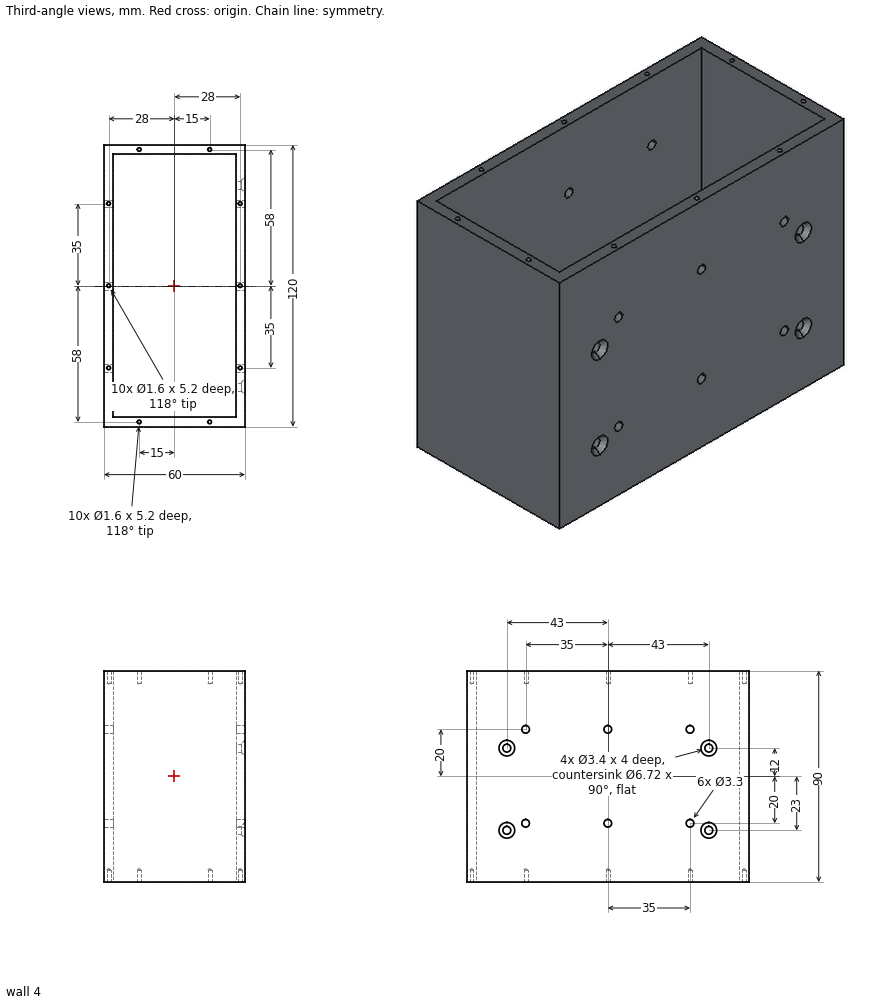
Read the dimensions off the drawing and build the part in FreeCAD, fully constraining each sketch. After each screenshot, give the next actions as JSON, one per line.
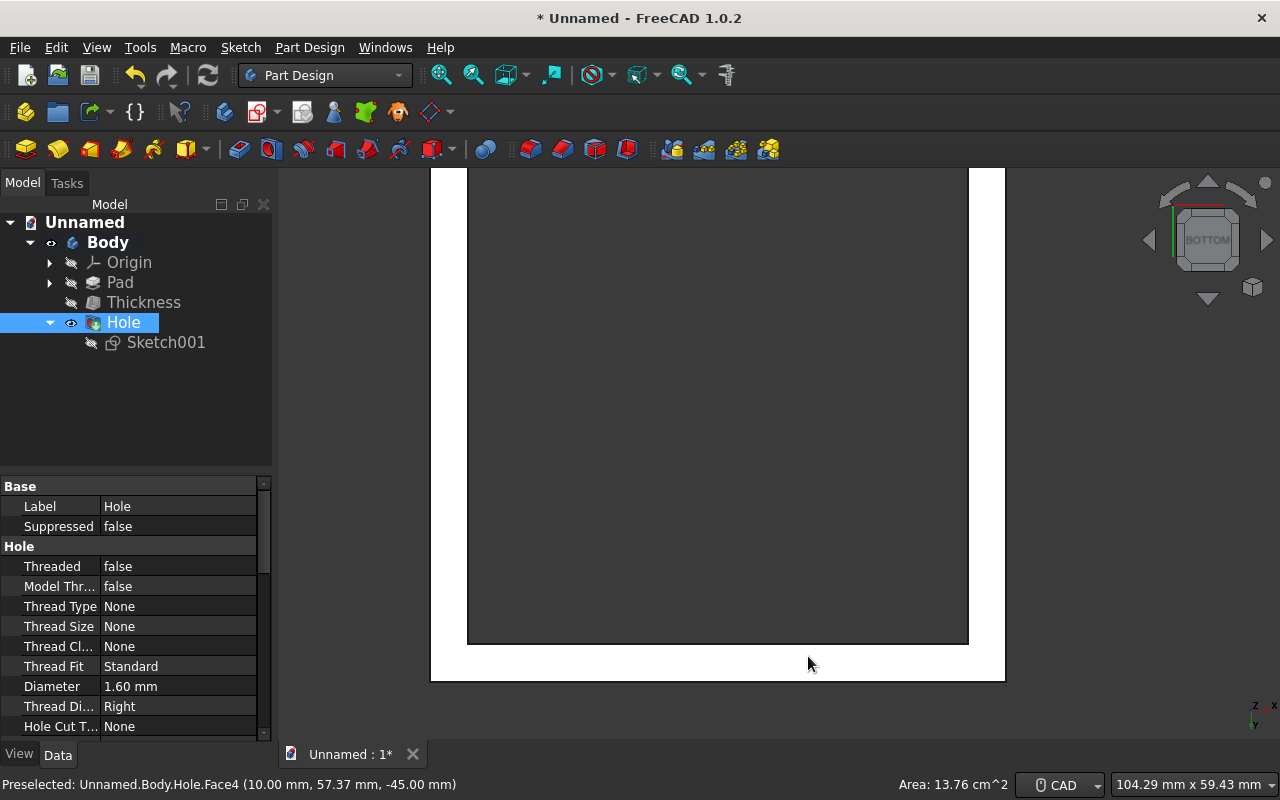
{"action": "left_click", "coordinate": [258, 112]}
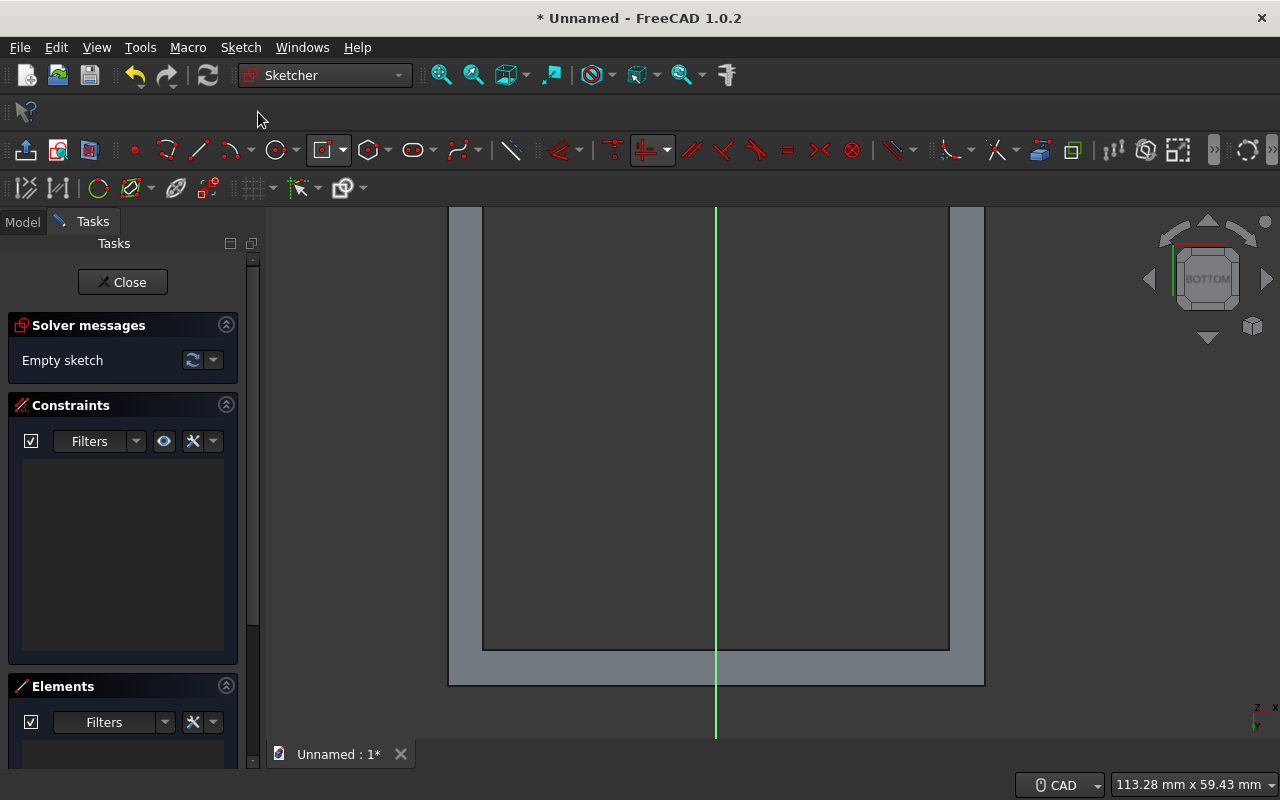
{"action": "scroll", "coordinate": [699, 613], "scroll_direction": "down", "scroll_amount": 6}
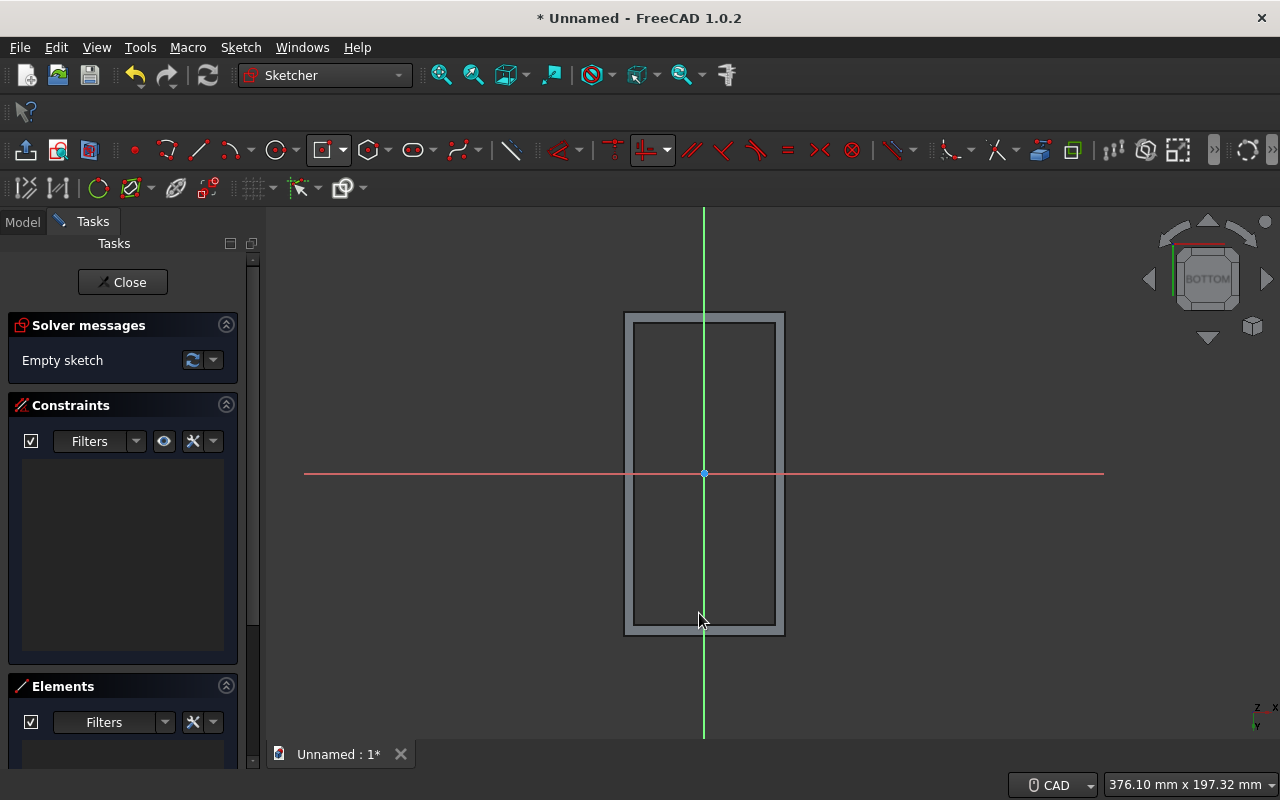
{"action": "left_click", "coordinate": [276, 150]}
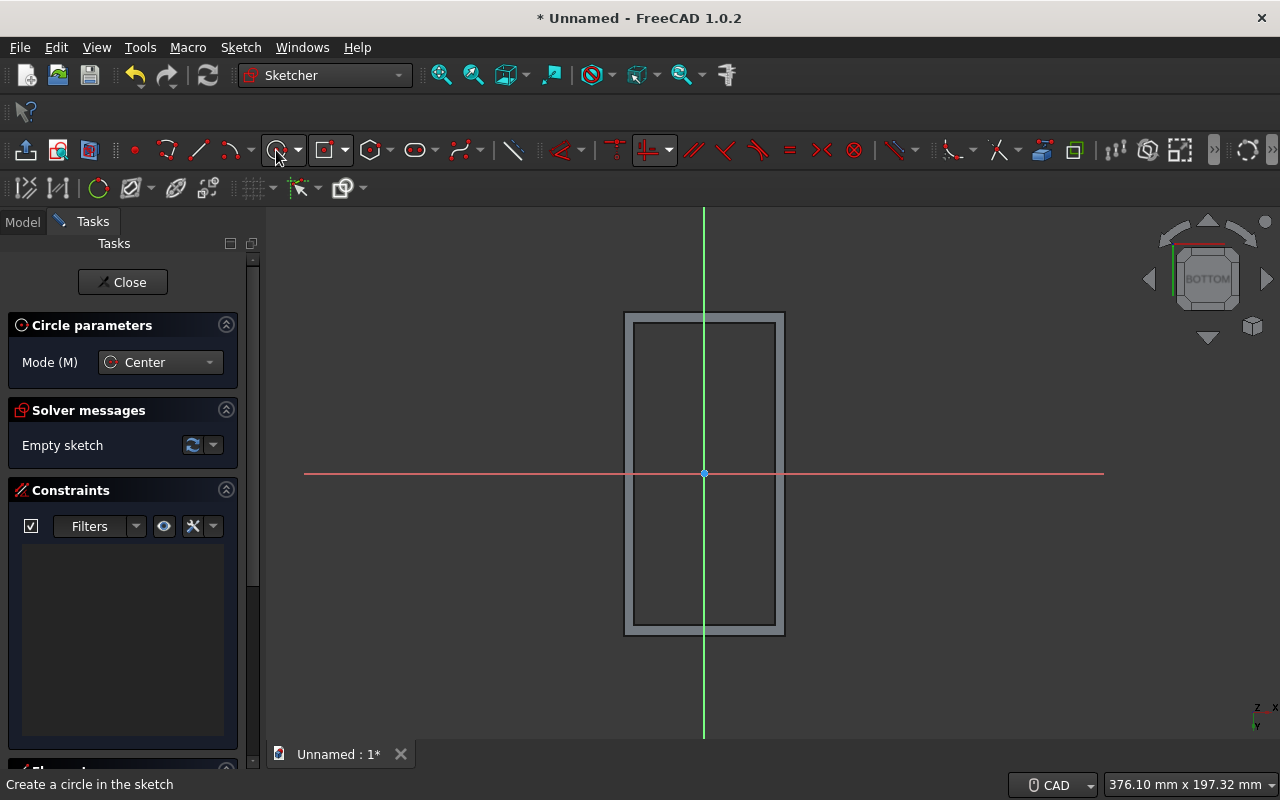
{"action": "scroll", "coordinate": [629, 474], "scroll_direction": "up", "scroll_amount": 12}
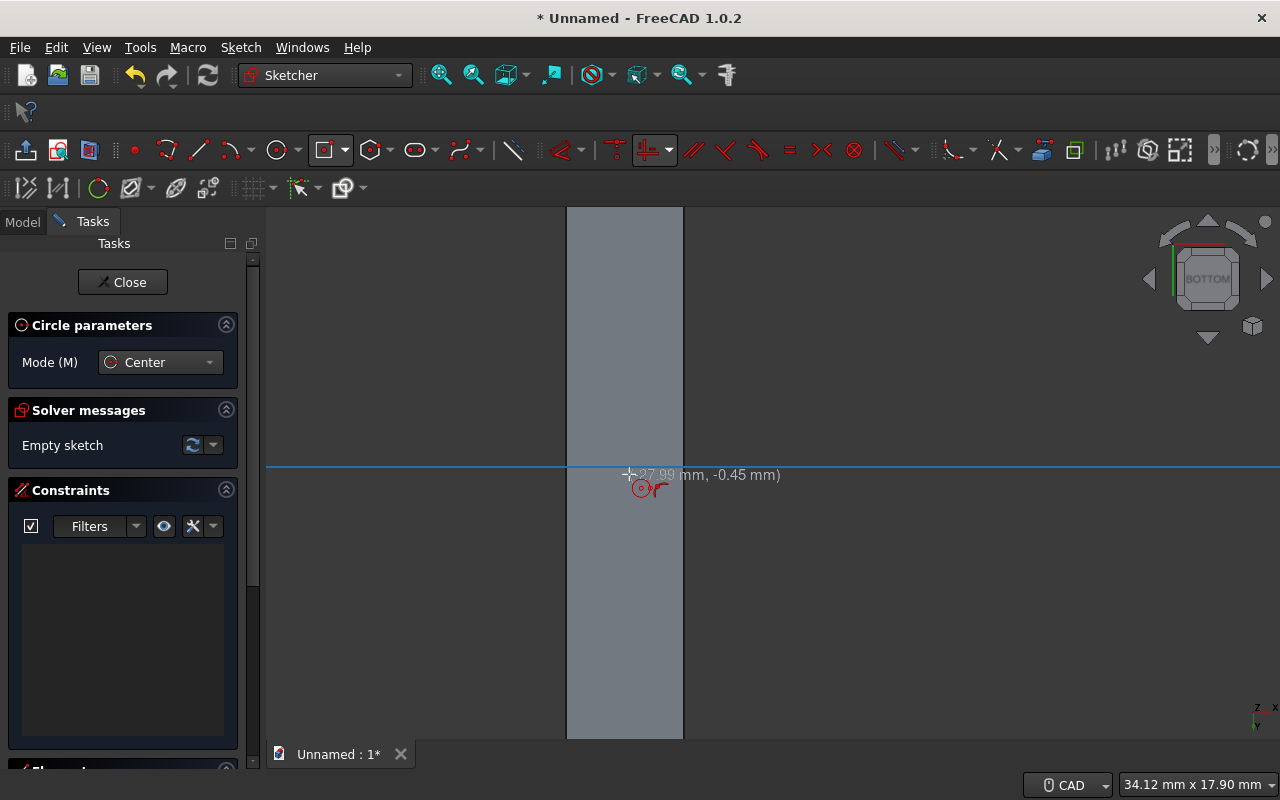
{"action": "scroll", "coordinate": [629, 474], "scroll_direction": "down", "scroll_amount": 12}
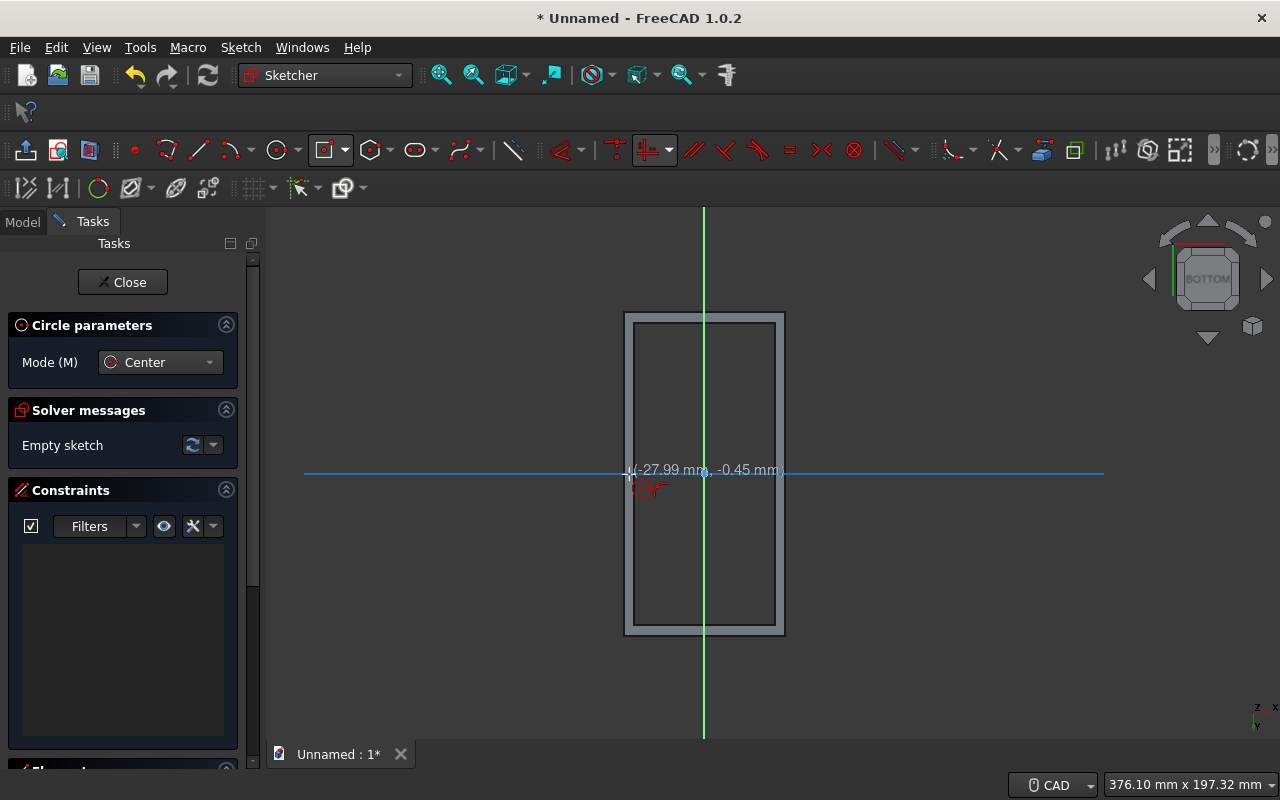
{"action": "left_click", "coordinate": [629, 474]}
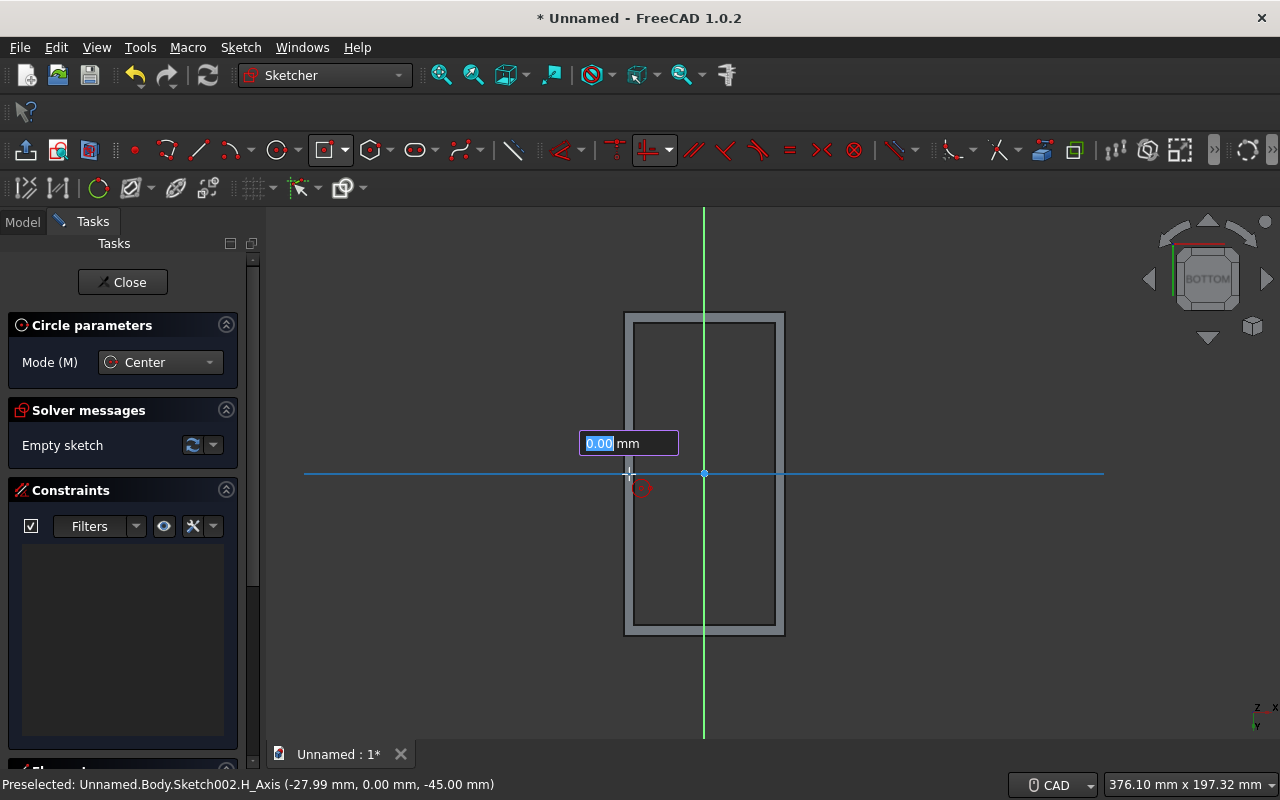
{"action": "scroll", "coordinate": [628, 476], "scroll_direction": "up", "scroll_amount": 11}
{"action": "mouse_move", "coordinate": [627, 470]}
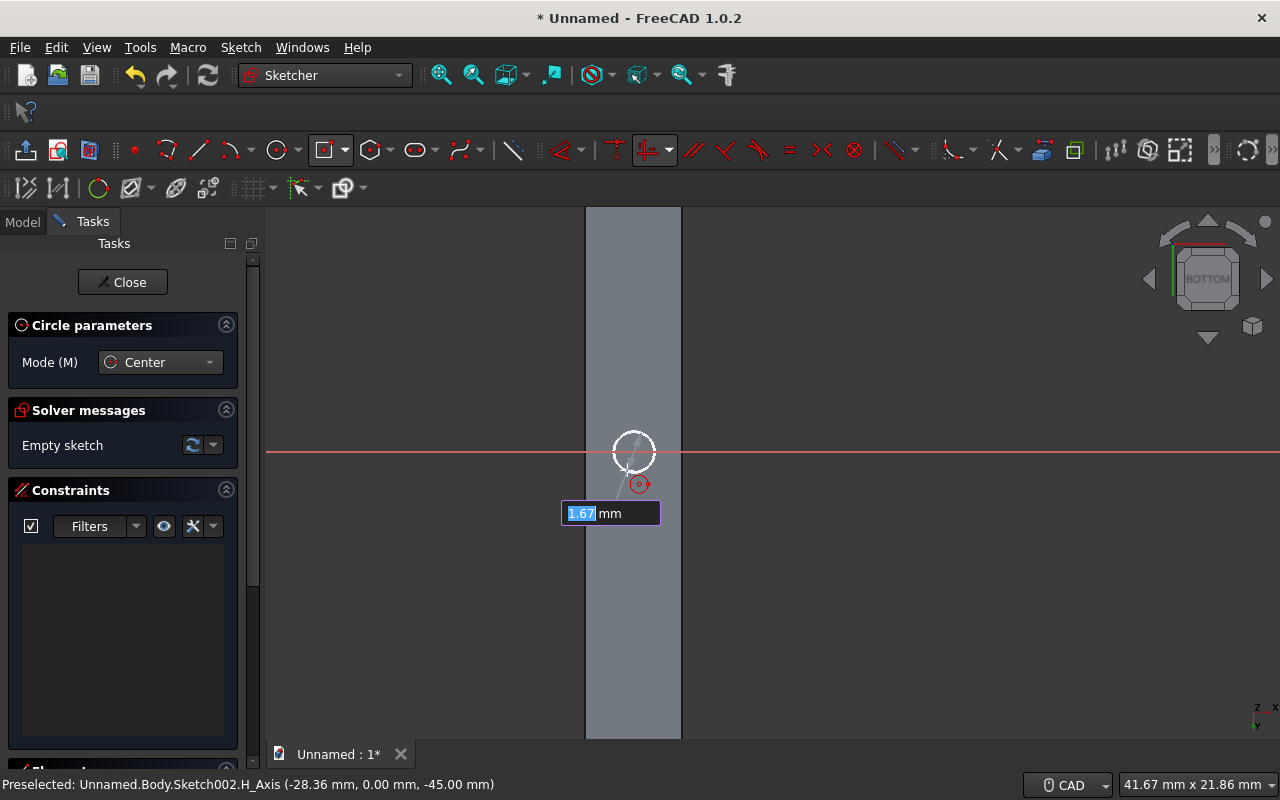
{"action": "type", "text": "1.6"}
{"action": "key", "text": "Return"}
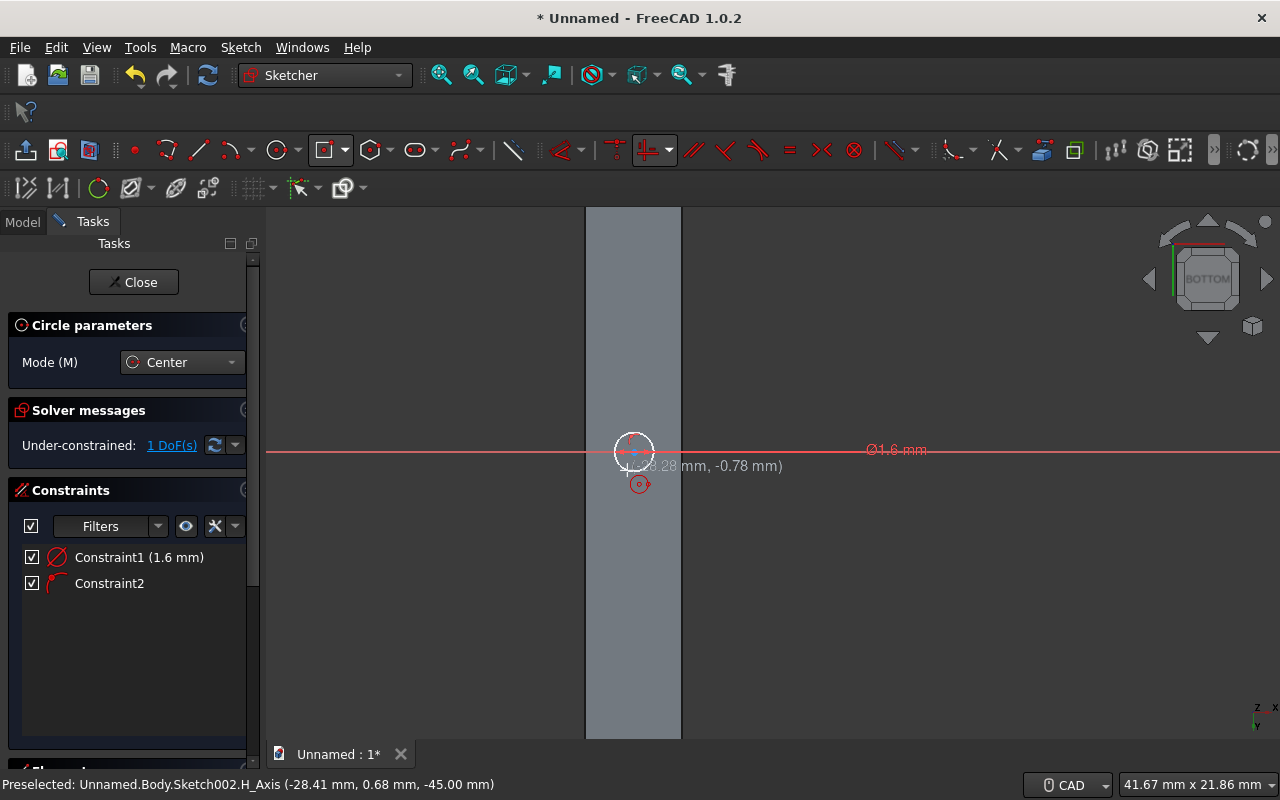
{"action": "scroll", "coordinate": [628, 476], "scroll_direction": "down", "scroll_amount": 11}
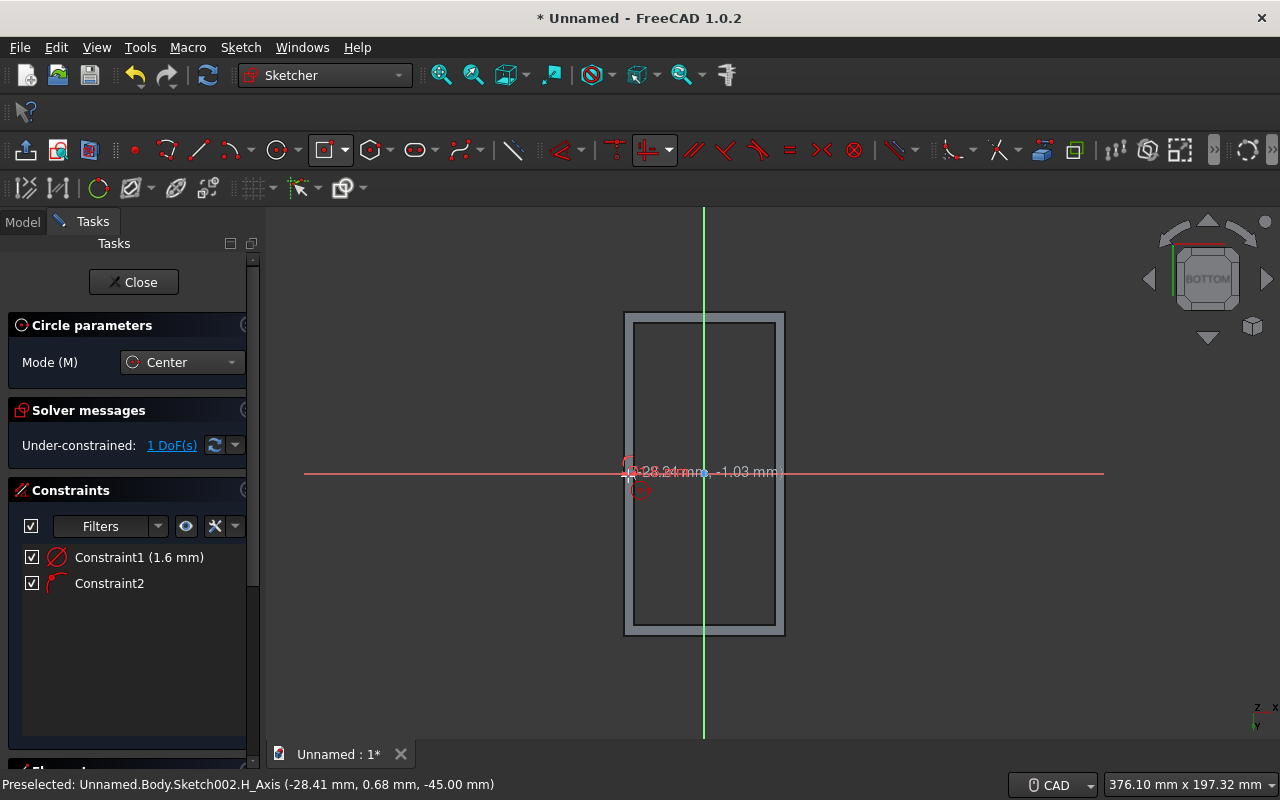
{"action": "scroll", "coordinate": [780, 474], "scroll_direction": "up", "scroll_amount": 12}